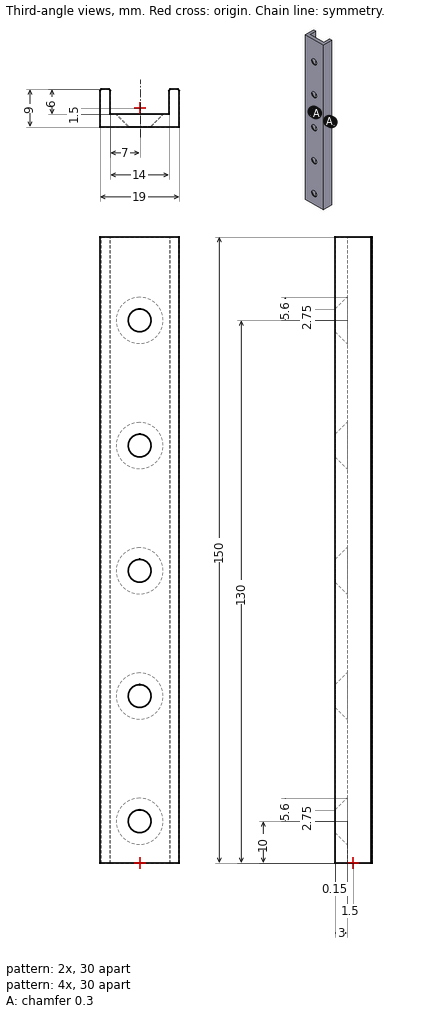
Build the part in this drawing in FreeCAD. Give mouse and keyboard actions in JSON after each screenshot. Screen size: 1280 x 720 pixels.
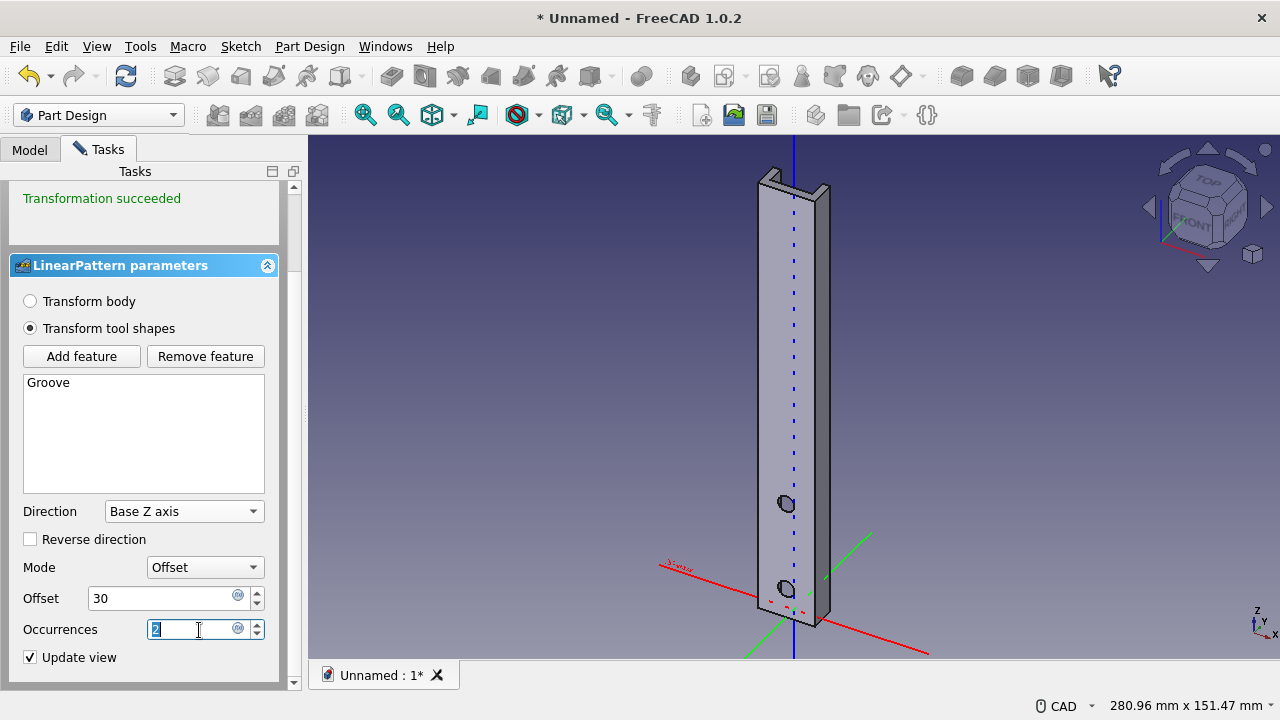
{"action": "type", "text": "2"}
{"action": "key", "text": "Tab"}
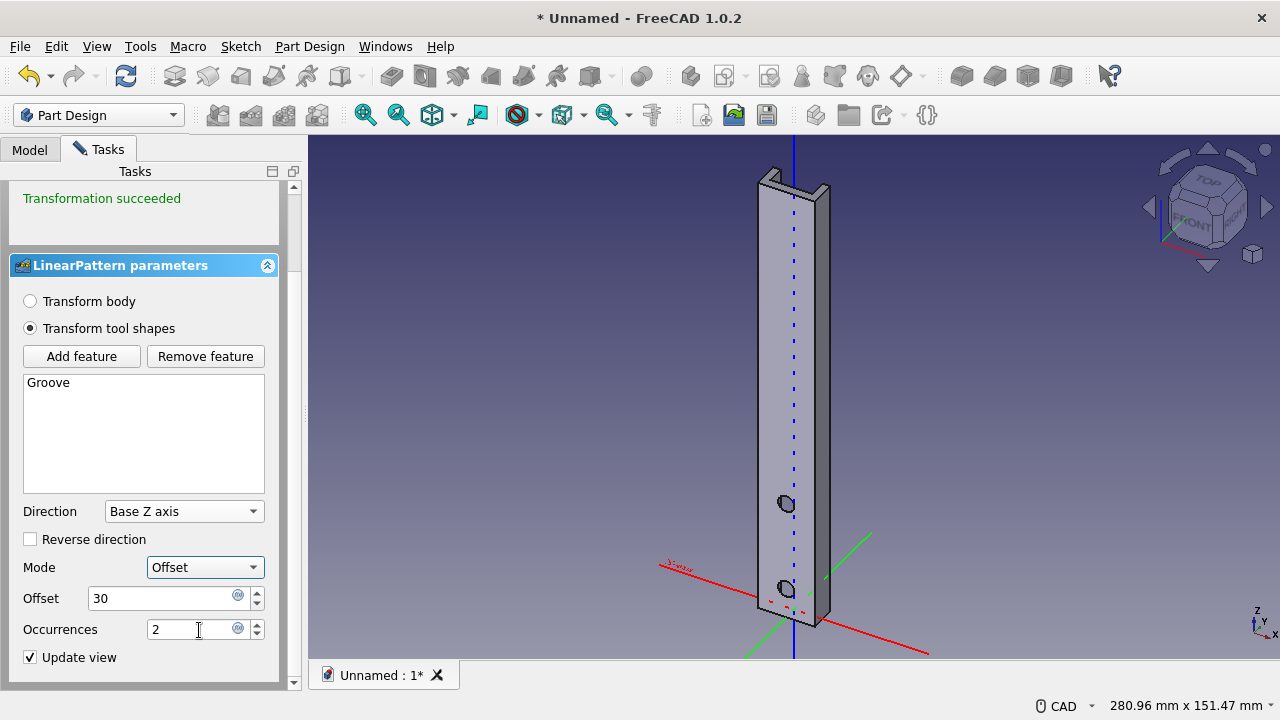
{"action": "scroll", "coordinate": [294, 436], "scroll_direction": "up", "scroll_amount": 3}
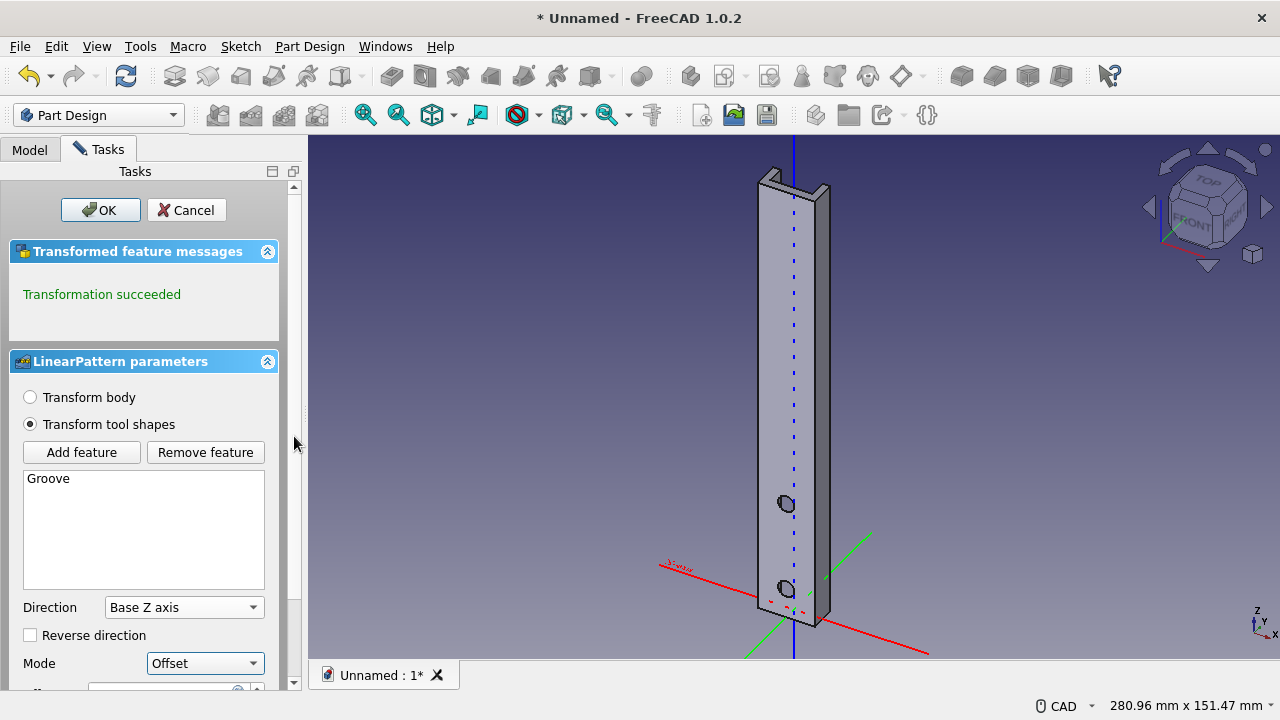
{"action": "left_click", "coordinate": [101, 210]}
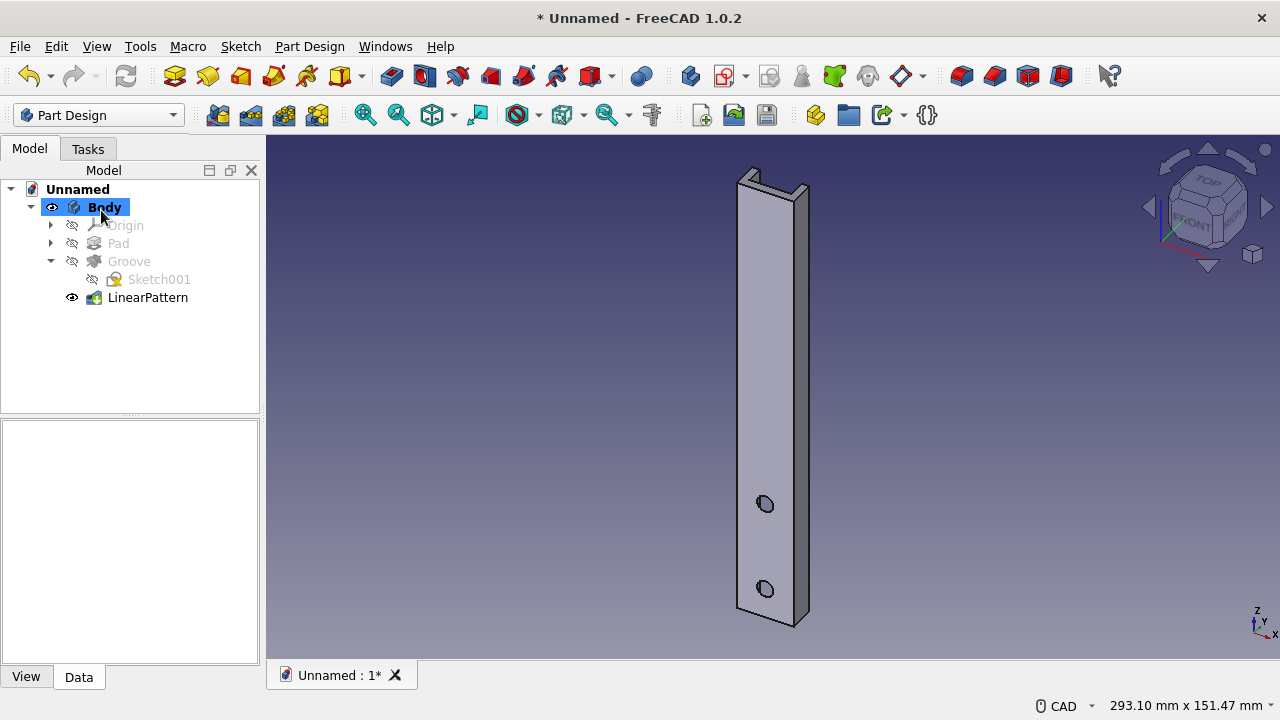
{"action": "left_click", "coordinate": [117, 261]}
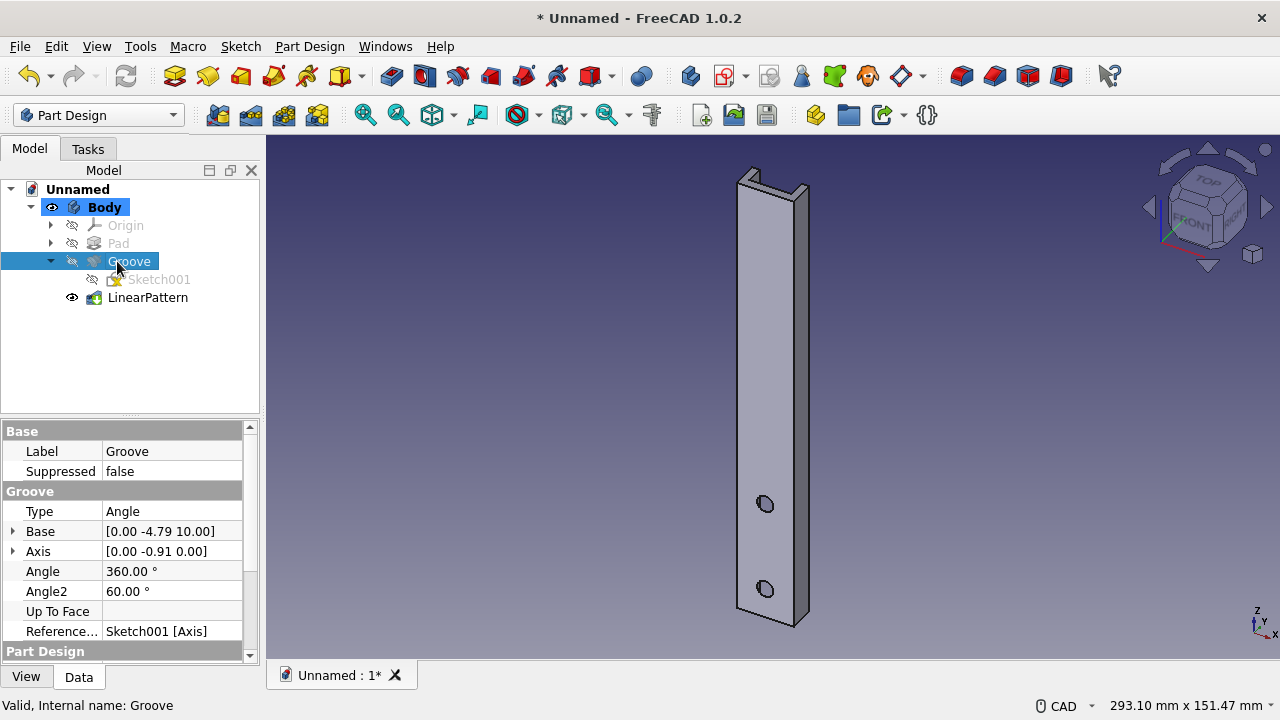
{"action": "left_click", "coordinate": [251, 116]}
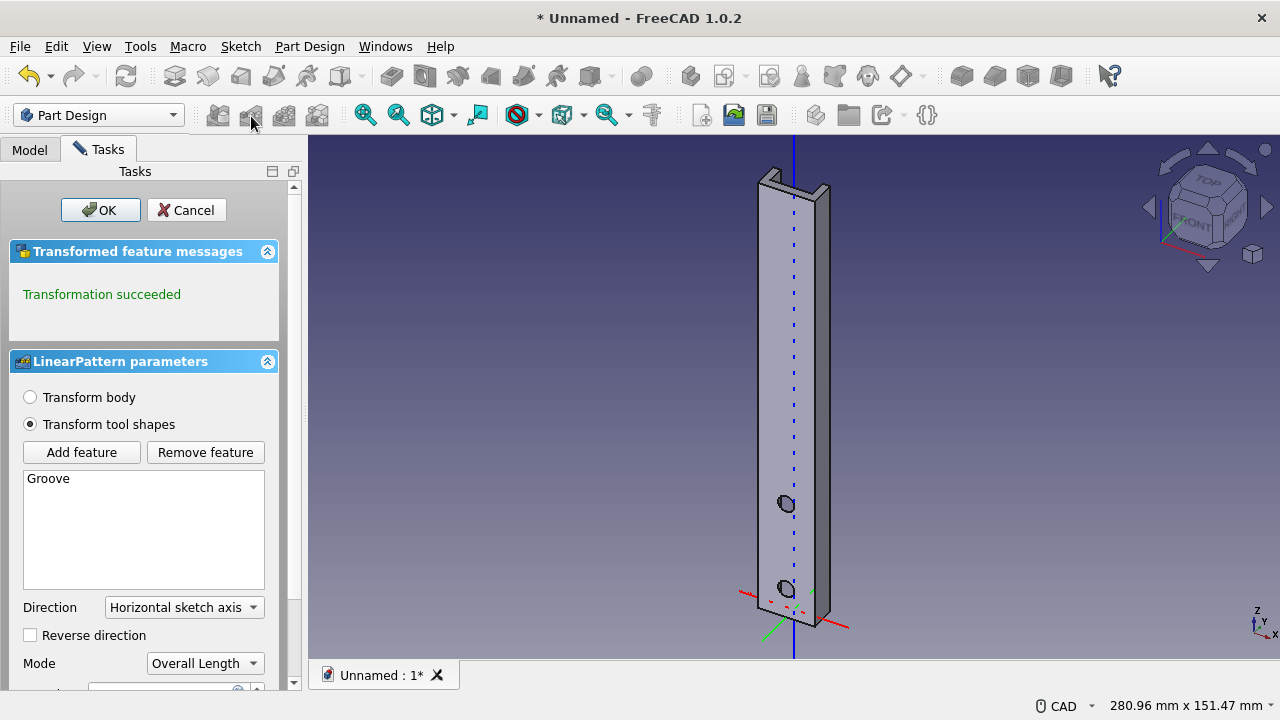
{"action": "left_click", "coordinate": [185, 608]}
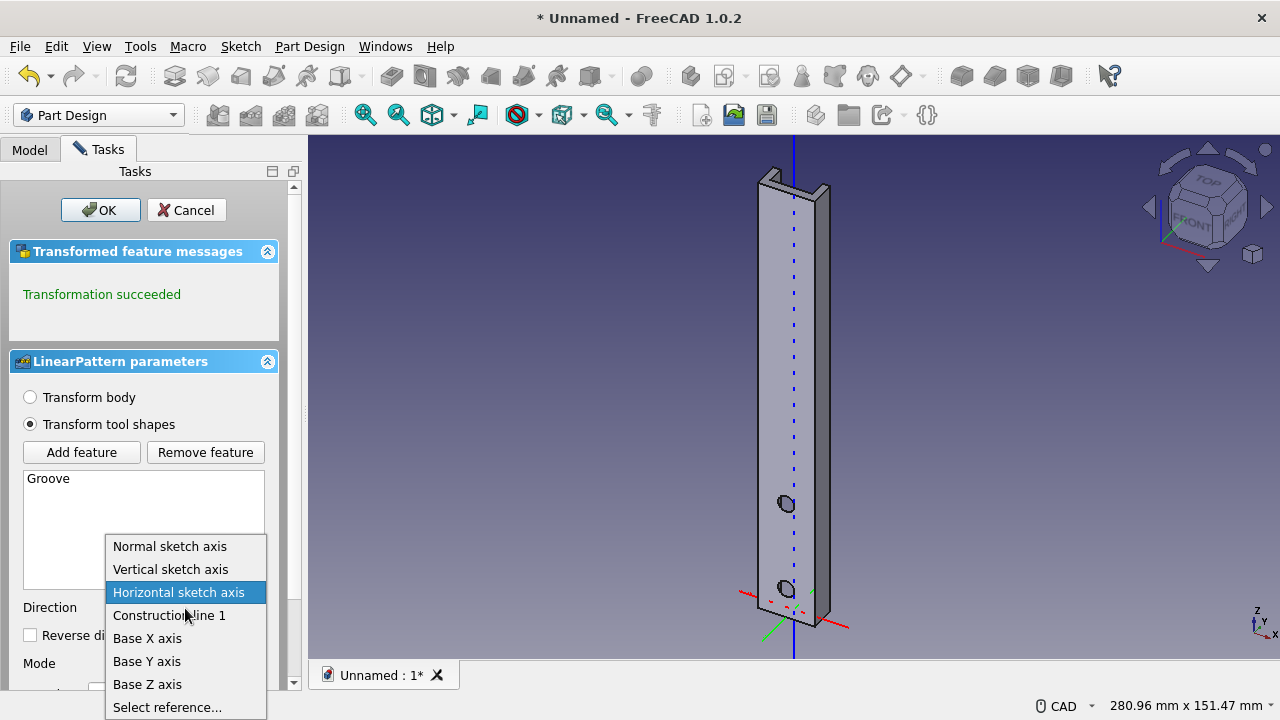
{"action": "left_click", "coordinate": [184, 684]}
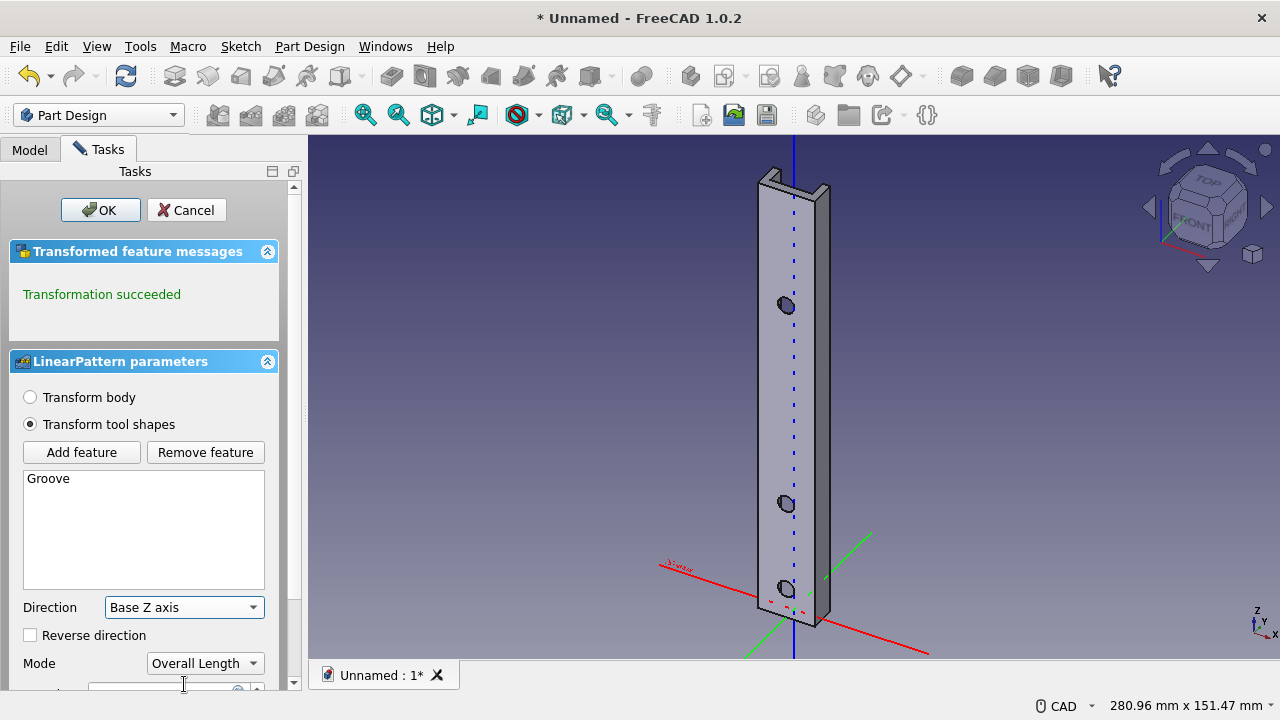
{"action": "left_click", "coordinate": [206, 664]}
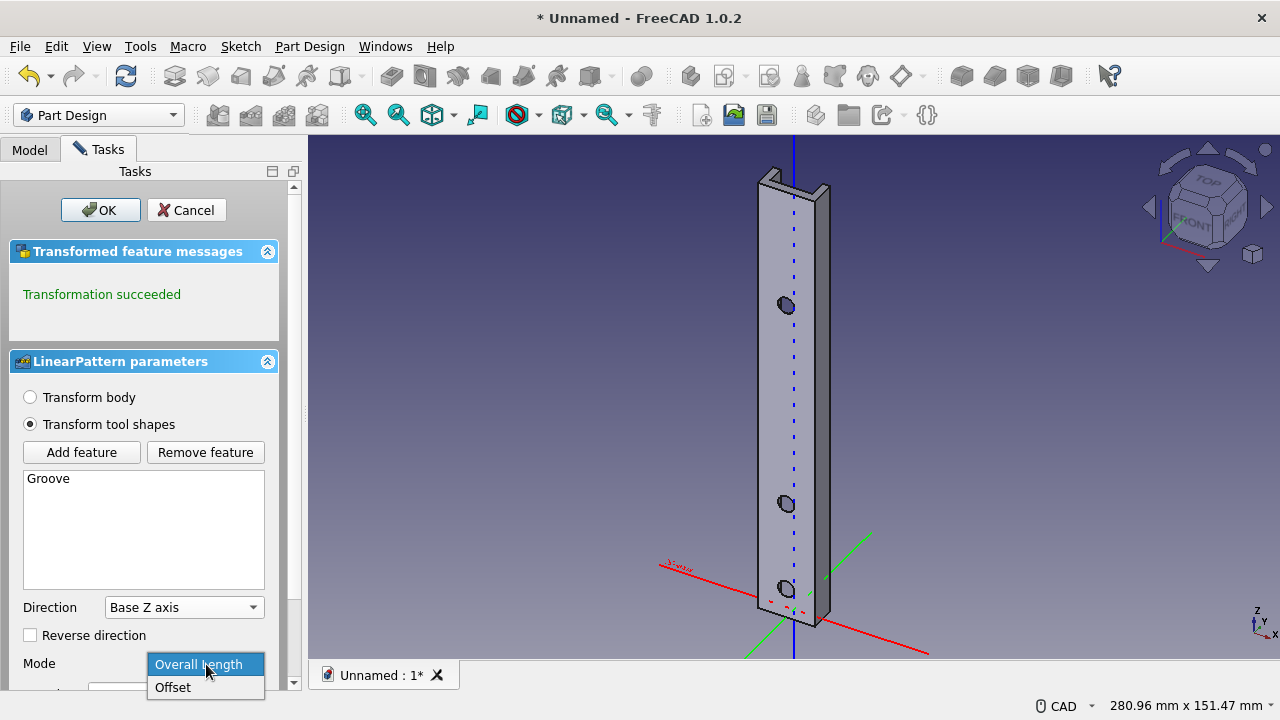
{"action": "left_click", "coordinate": [204, 688]}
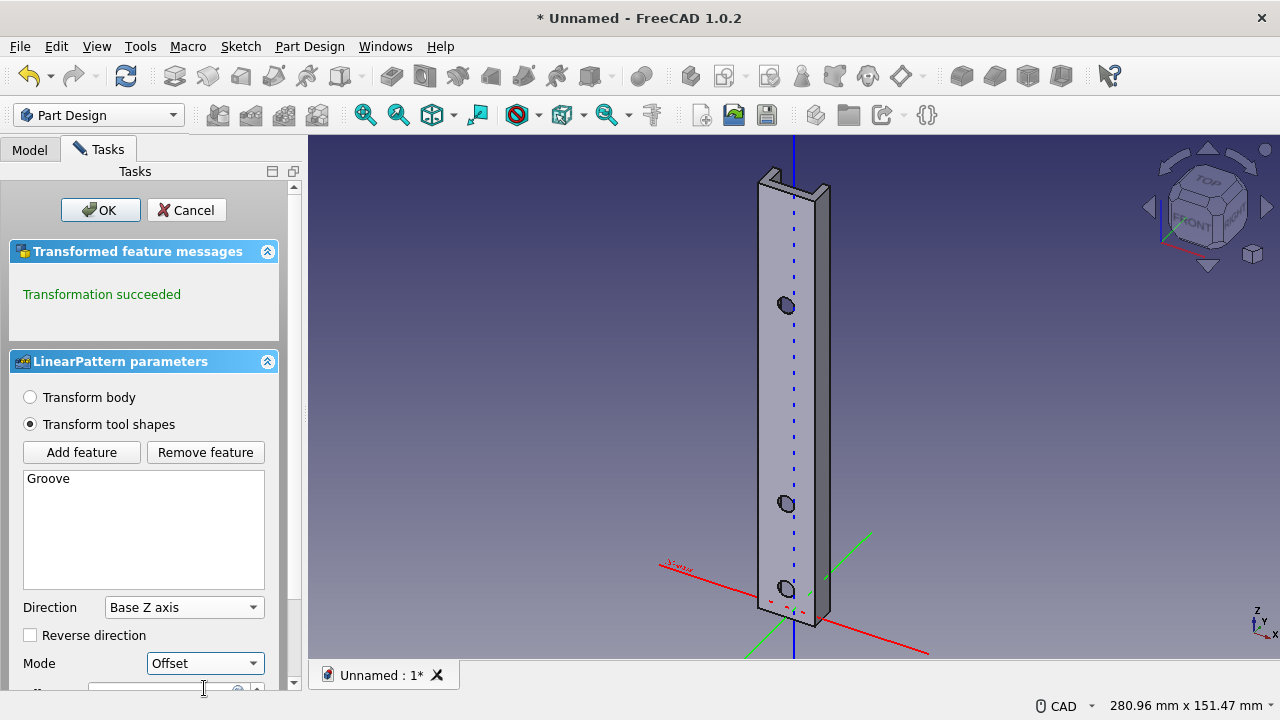
{"action": "scroll", "coordinate": [294, 436], "scroll_direction": "down", "scroll_amount": 2}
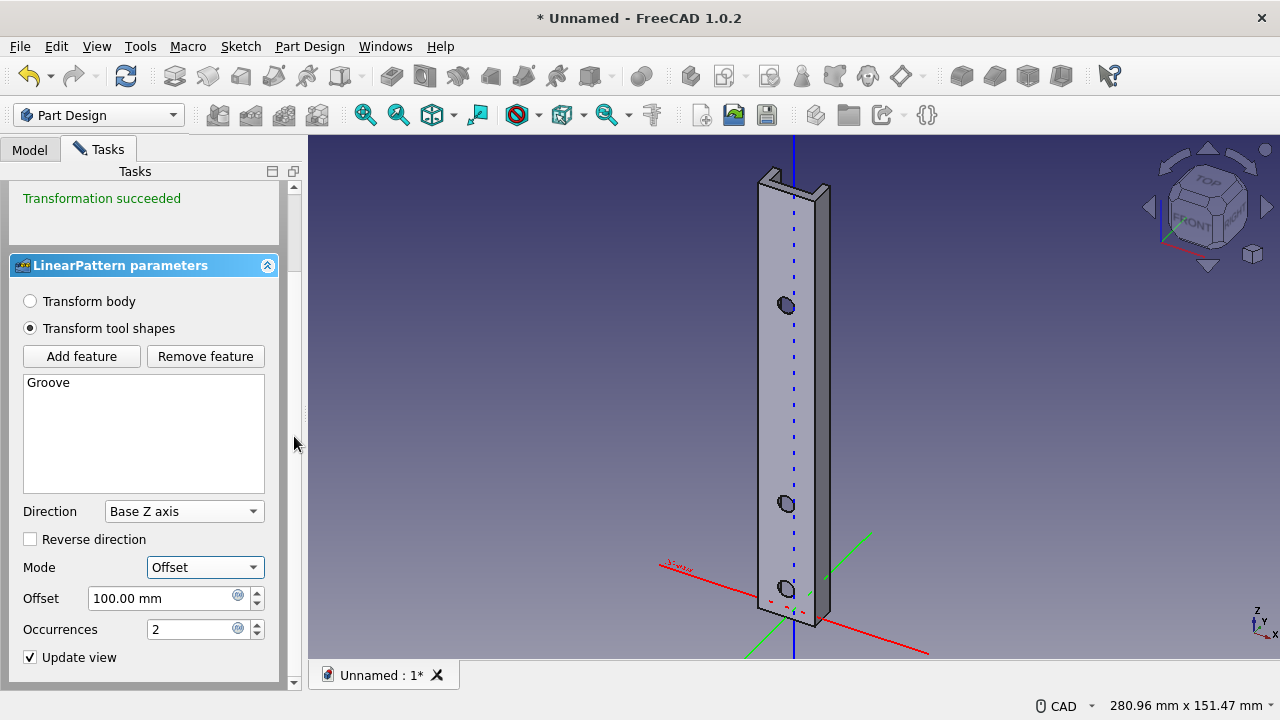
{"action": "triple_click", "coordinate": [170, 598]}